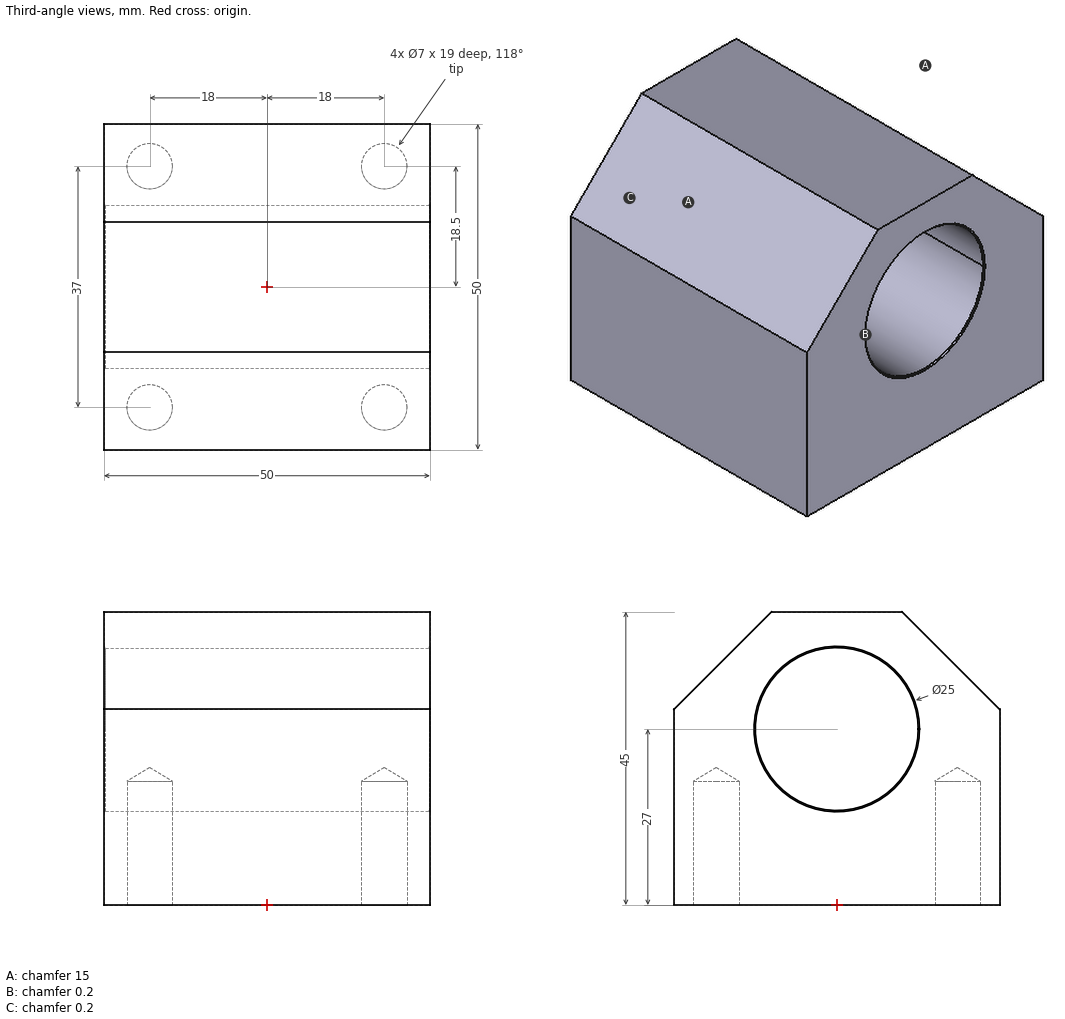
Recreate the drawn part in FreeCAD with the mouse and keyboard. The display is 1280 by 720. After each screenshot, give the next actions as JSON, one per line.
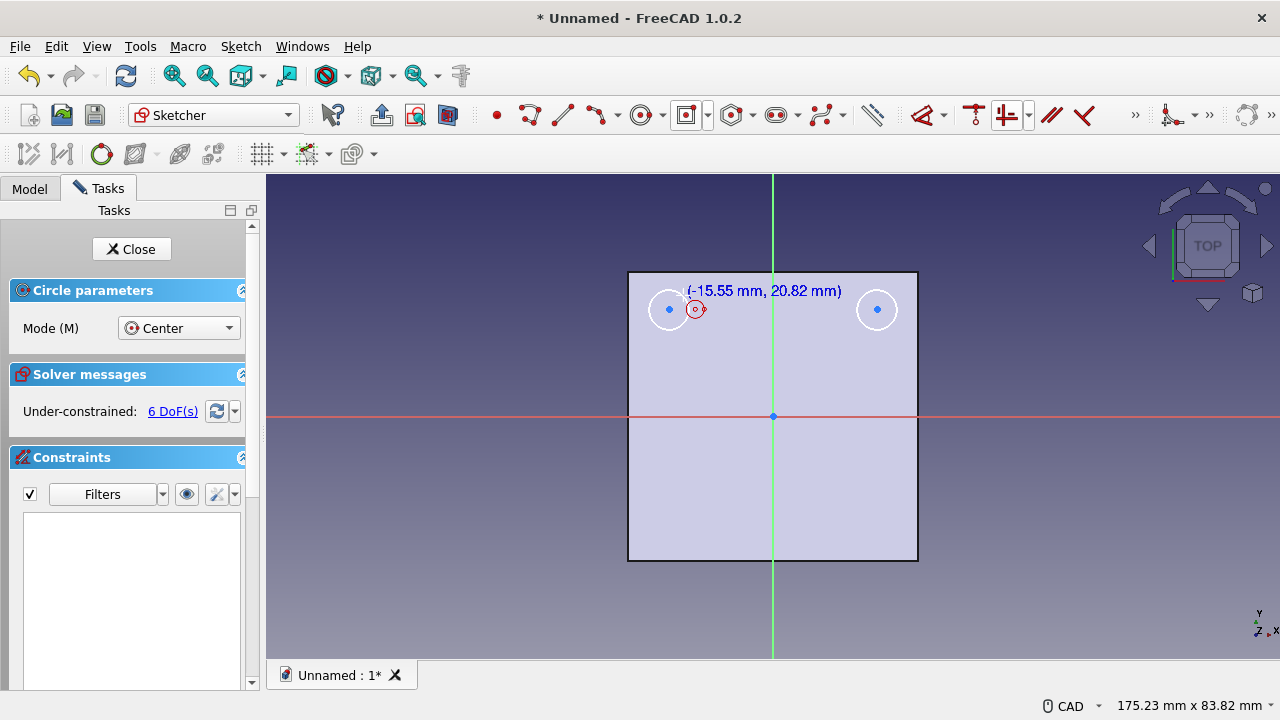
{"action": "left_click", "coordinate": [669, 524]}
{"action": "left_click", "coordinate": [683, 509]}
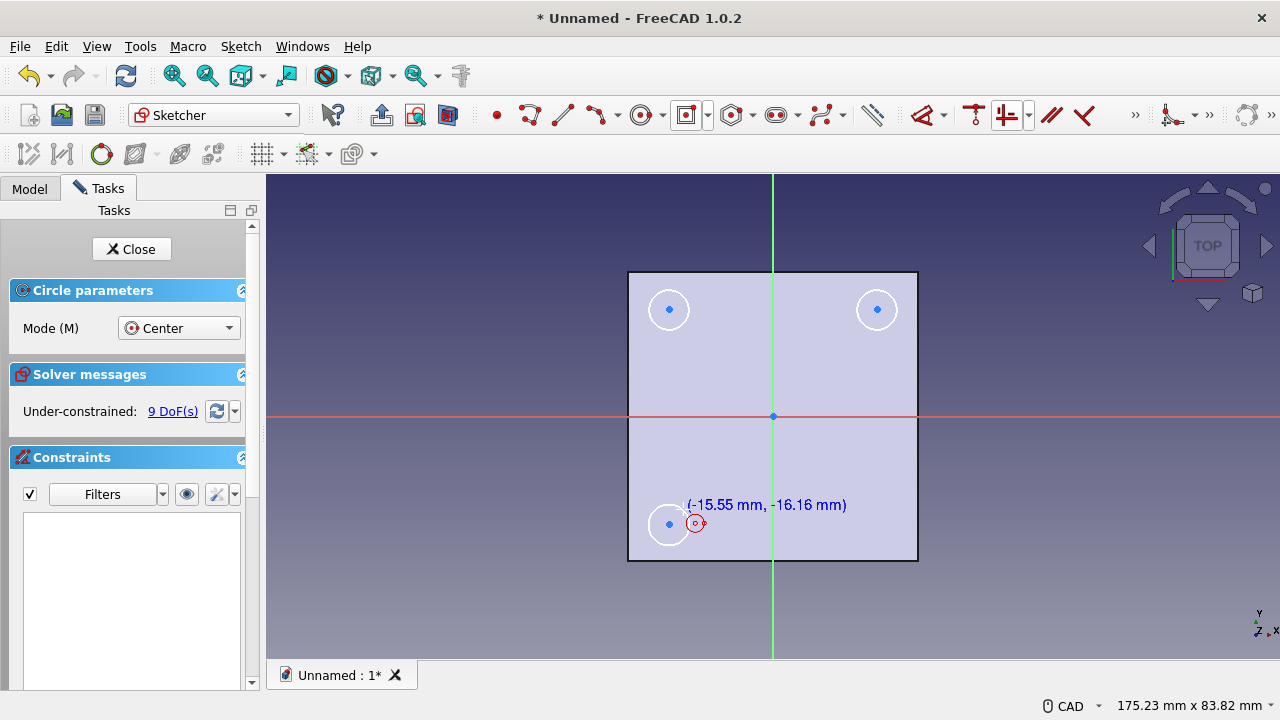
{"action": "left_click", "coordinate": [877, 524]}
{"action": "left_click", "coordinate": [891, 509]}
{"action": "key", "text": "Escape"}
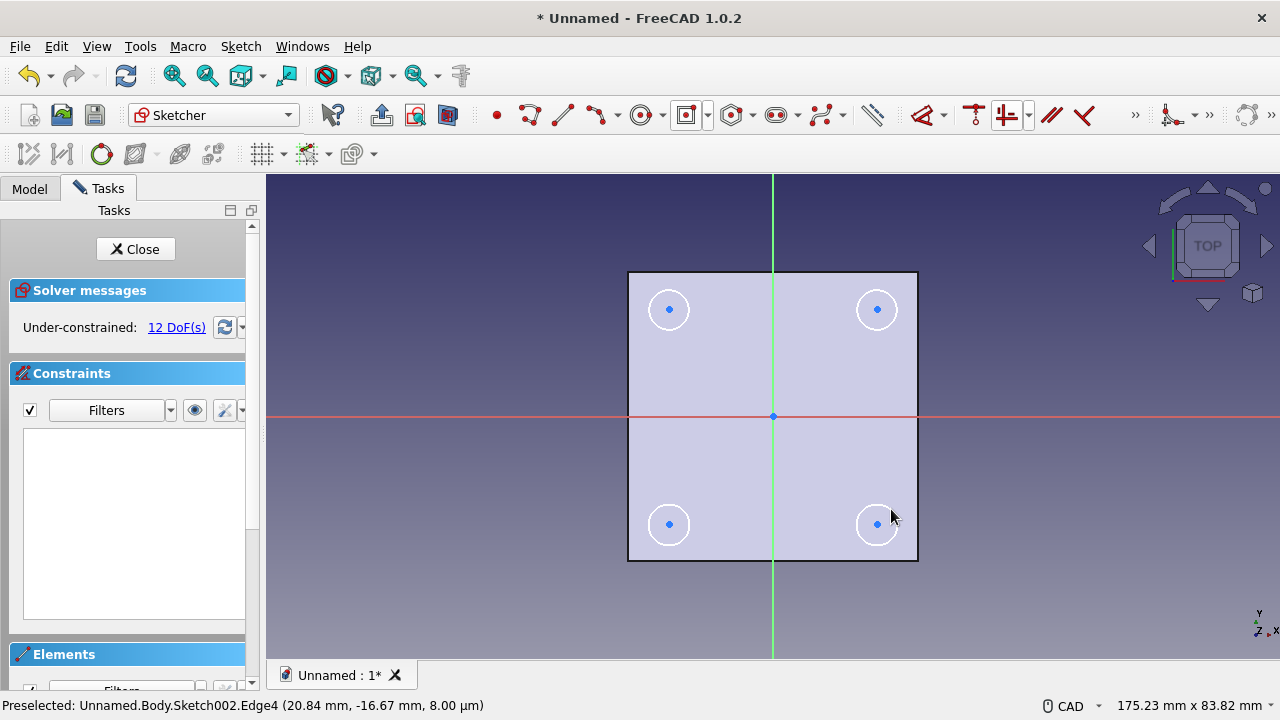
{"action": "left_click", "coordinate": [891, 296]}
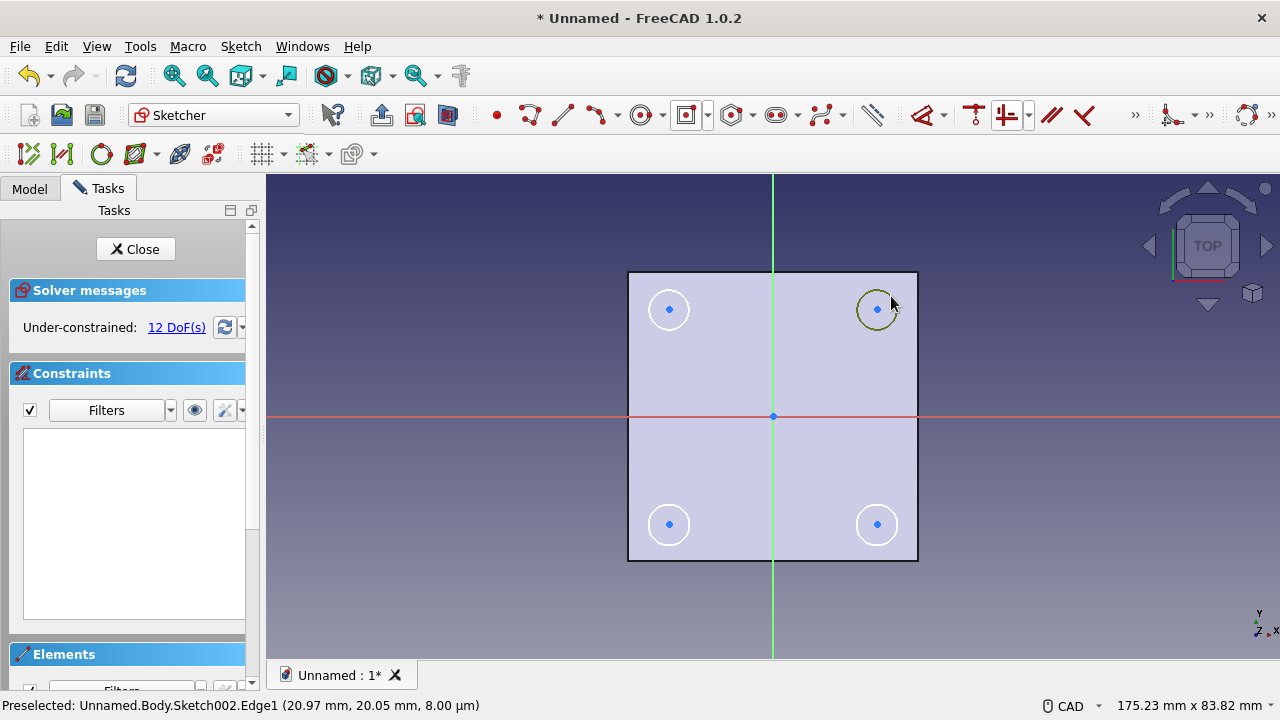
{"action": "left_click", "coordinate": [683, 296]}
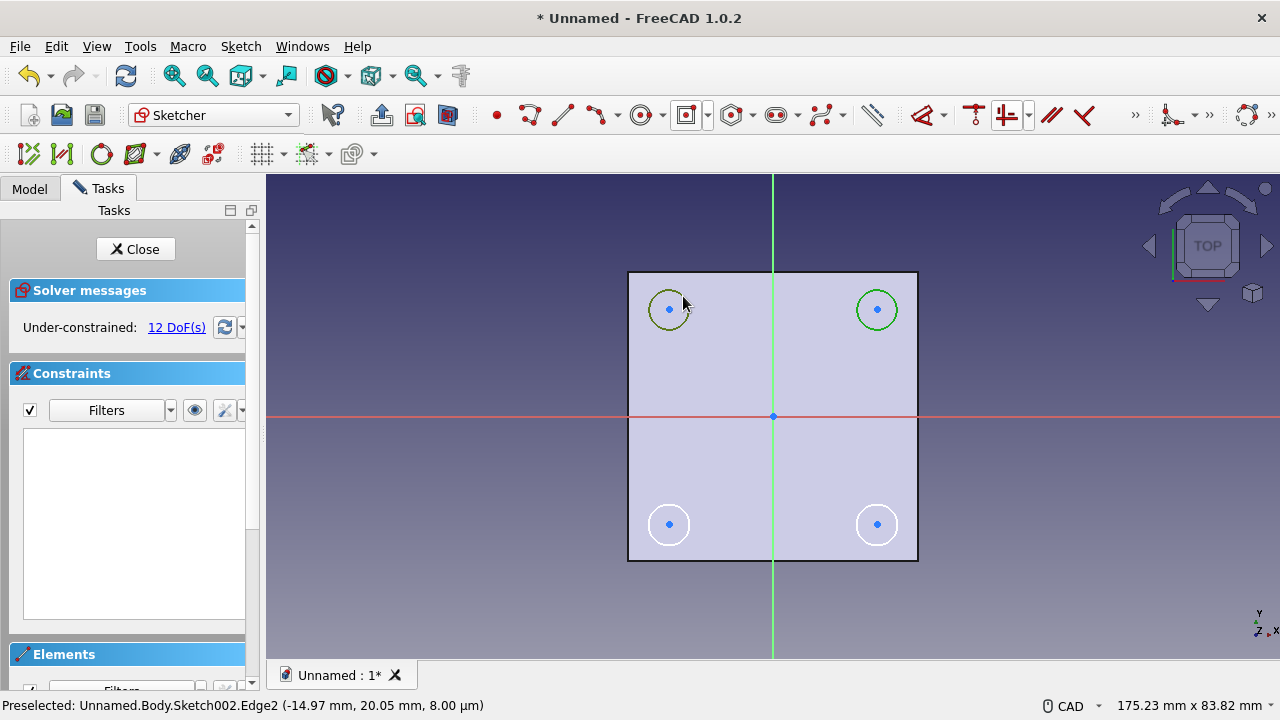
{"action": "left_click", "coordinate": [683, 510]}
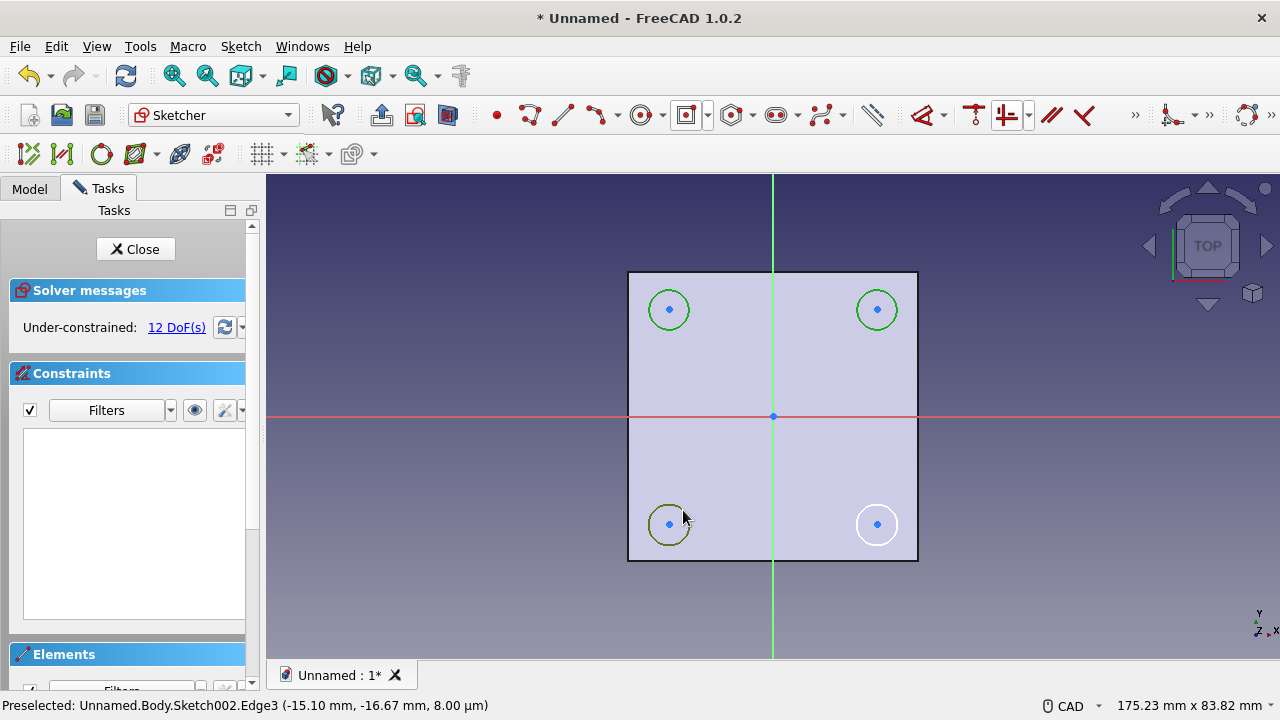
{"action": "left_click", "coordinate": [891, 510]}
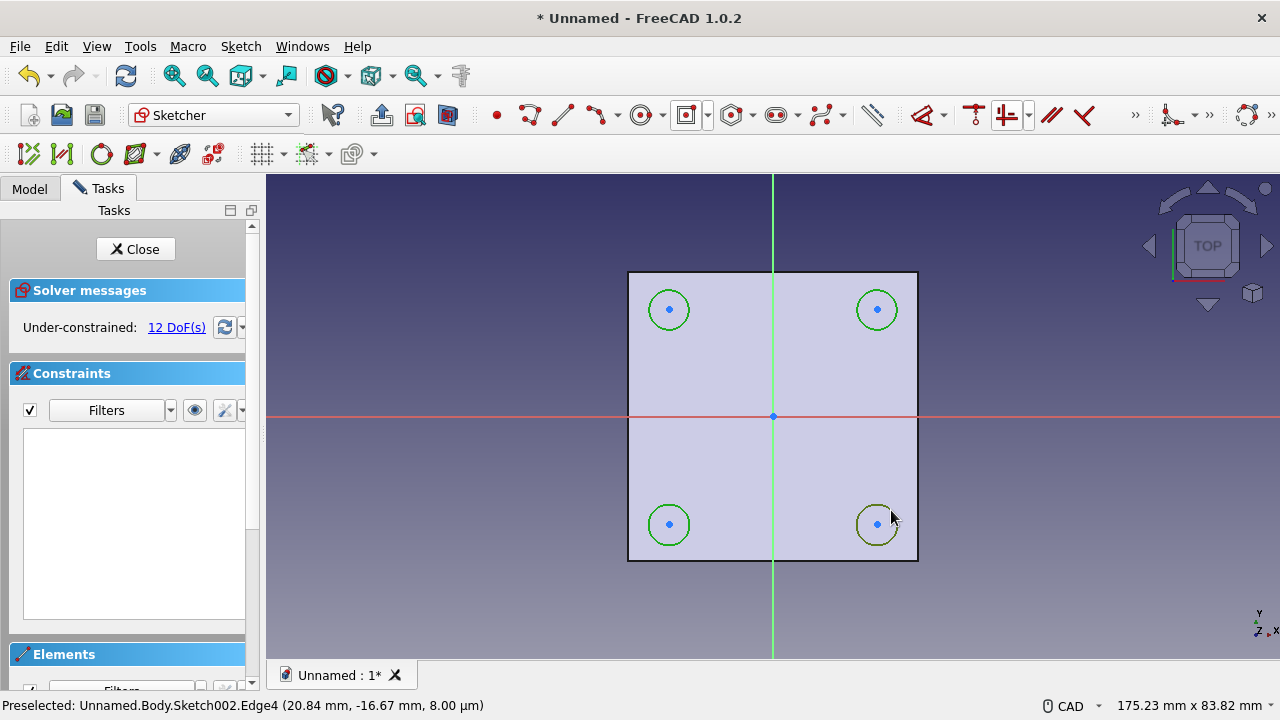
{"action": "key", "text": "e"}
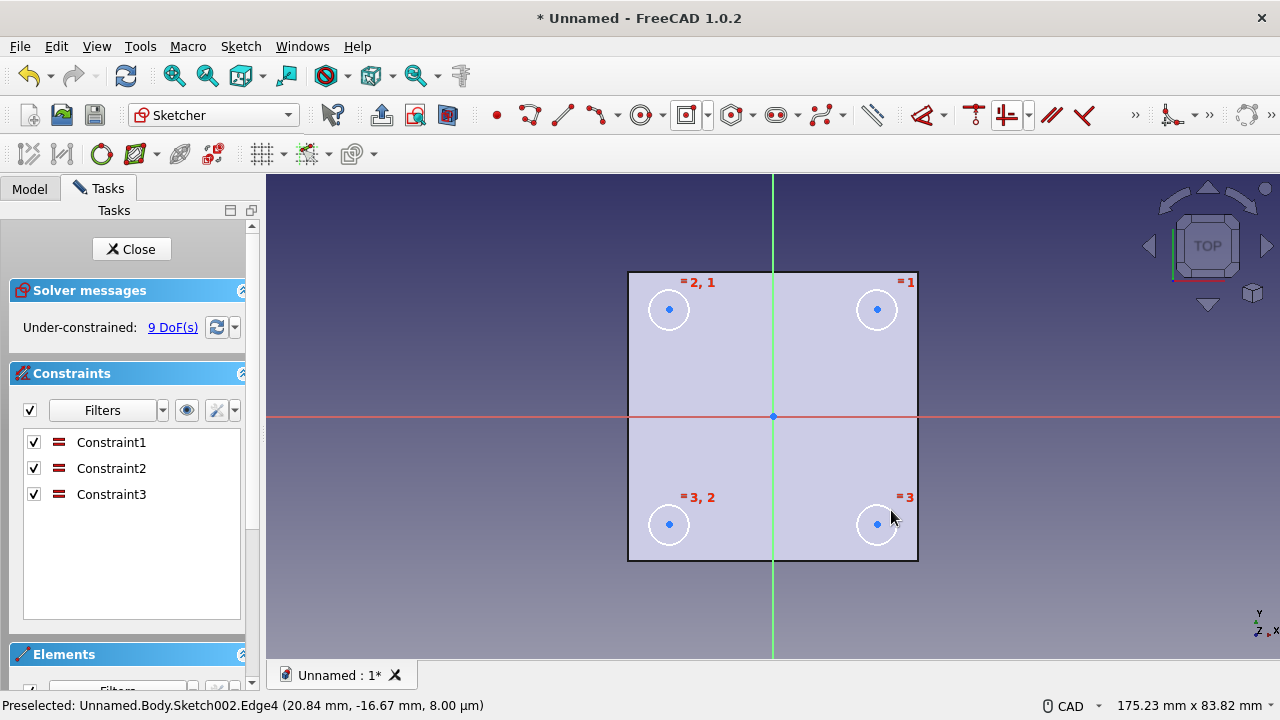
{"action": "left_click", "coordinate": [922, 116]}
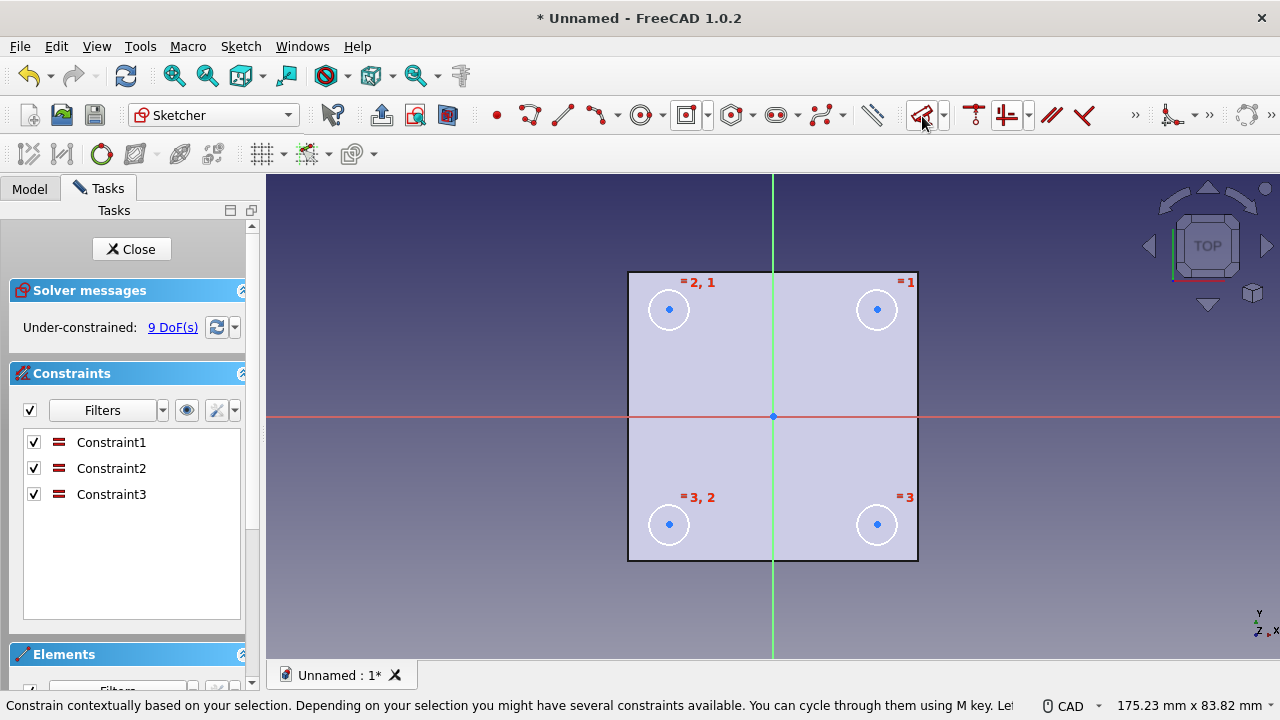
{"action": "left_click", "coordinate": [891, 296]}
{"action": "left_click", "coordinate": [914, 273]}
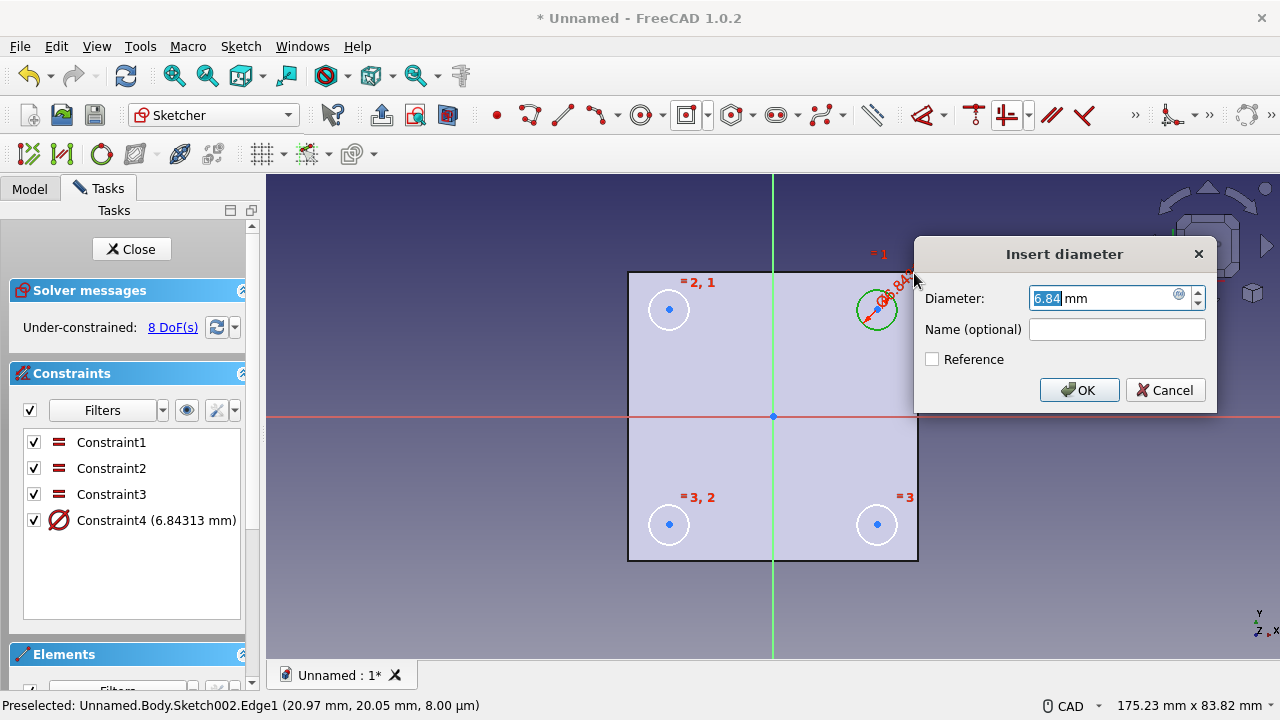
{"action": "type", "text": "7"}
{"action": "key", "text": "Return"}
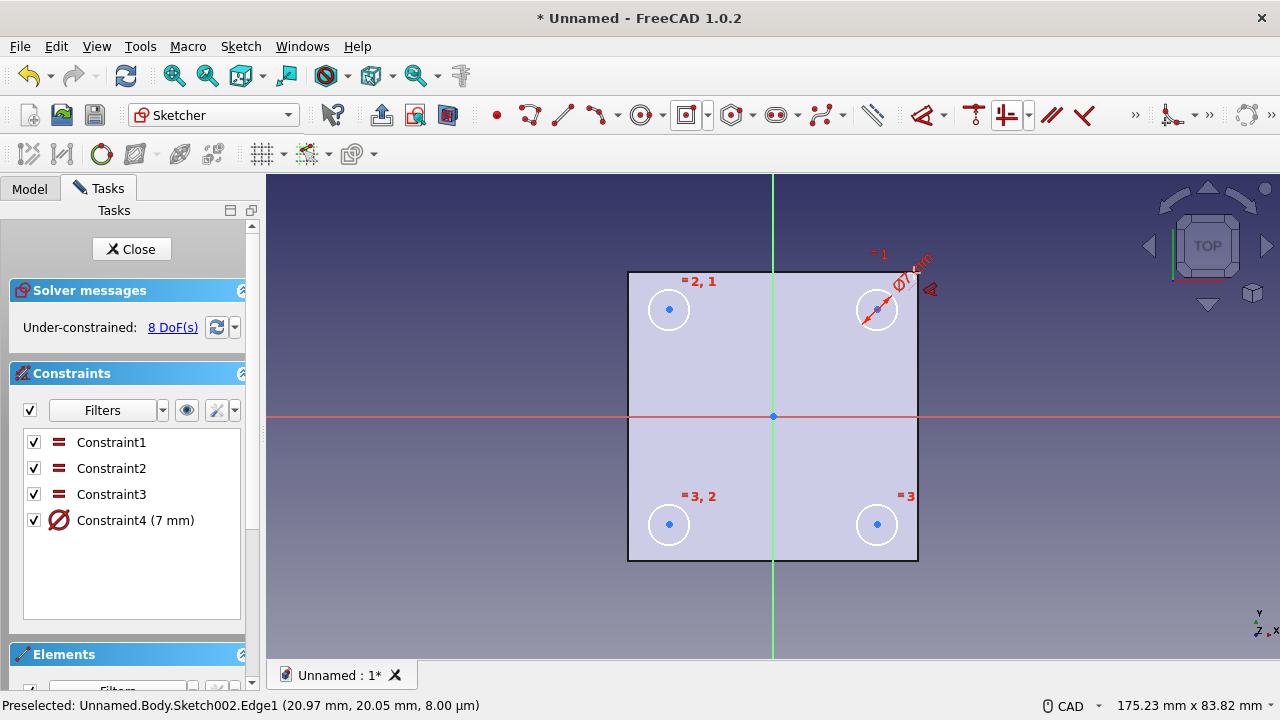
{"action": "left_click", "coordinate": [877, 310]}
{"action": "left_click", "coordinate": [825, 276]}